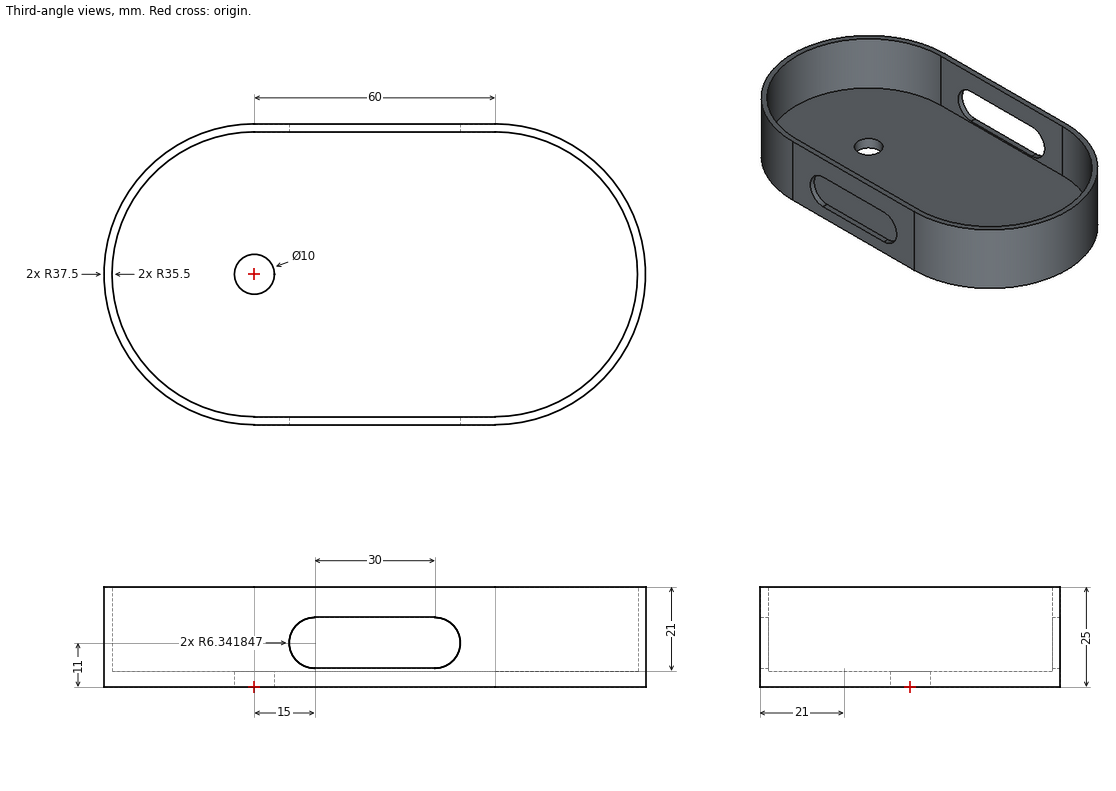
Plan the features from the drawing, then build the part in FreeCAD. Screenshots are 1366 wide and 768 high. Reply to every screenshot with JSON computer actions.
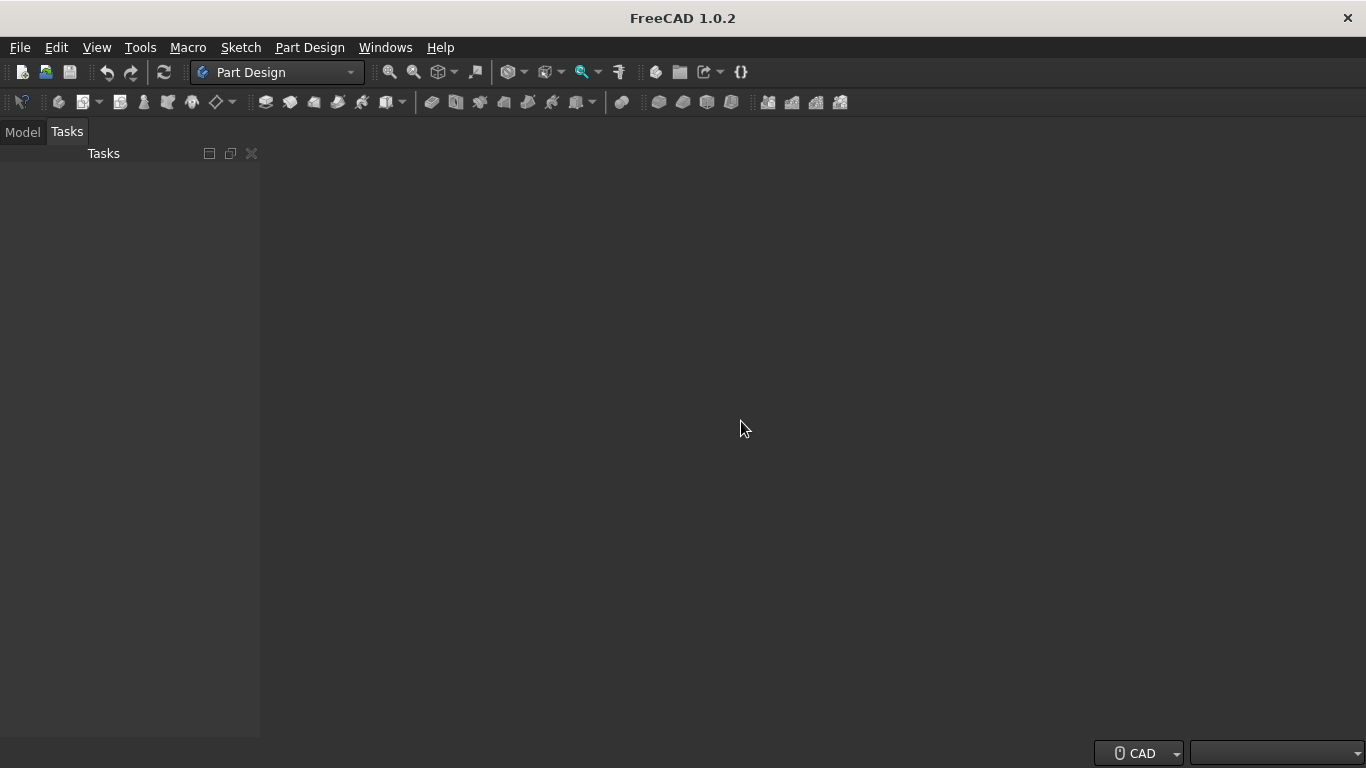
{"action": "left_click", "coordinate": [22, 72]}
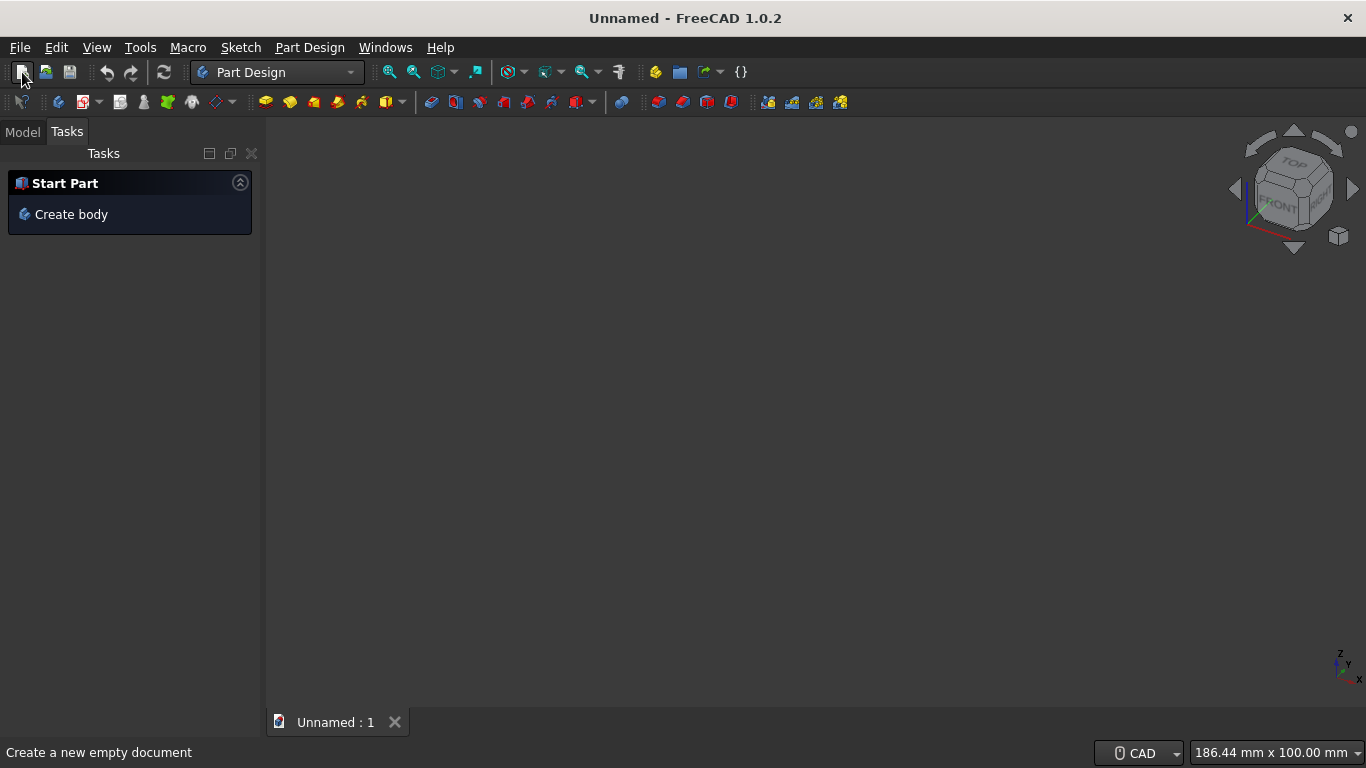
{"action": "left_click", "coordinate": [84, 102]}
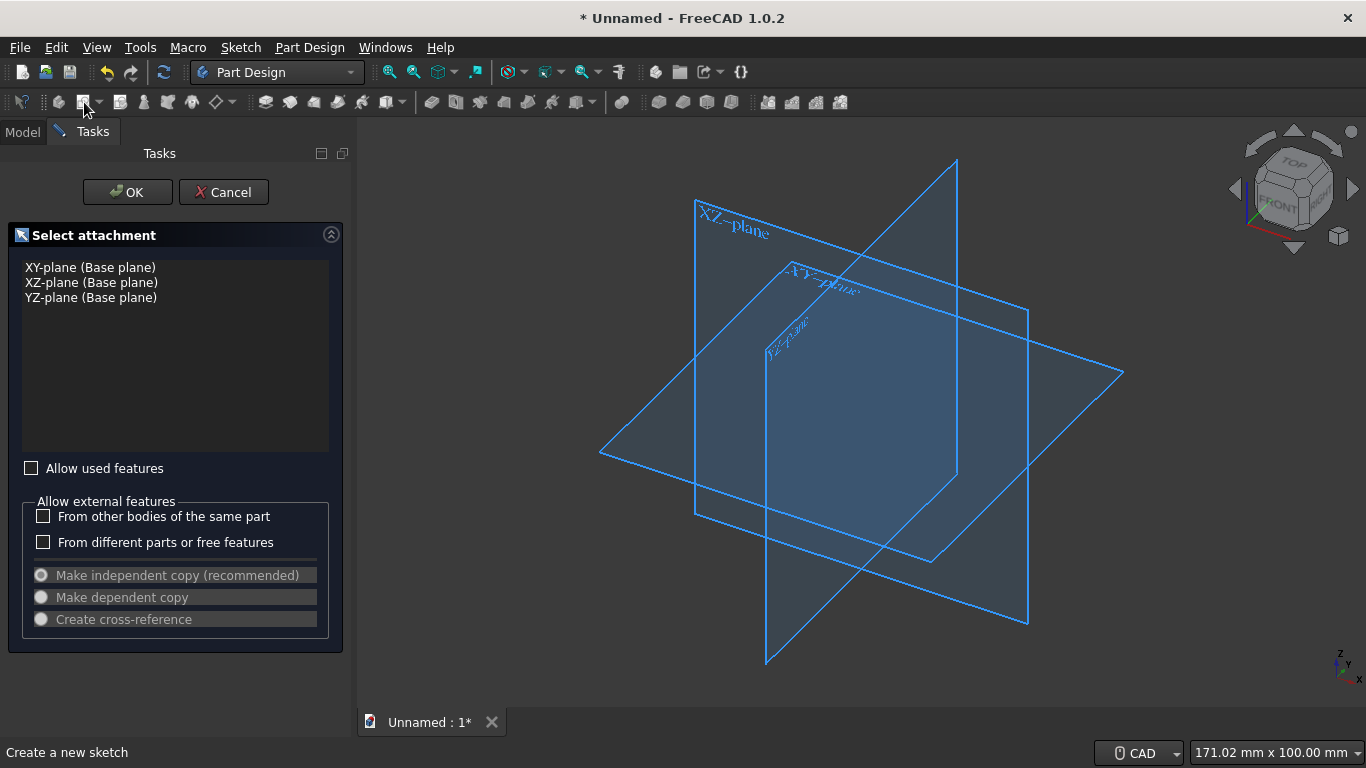
{"action": "left_click", "coordinate": [82, 268]}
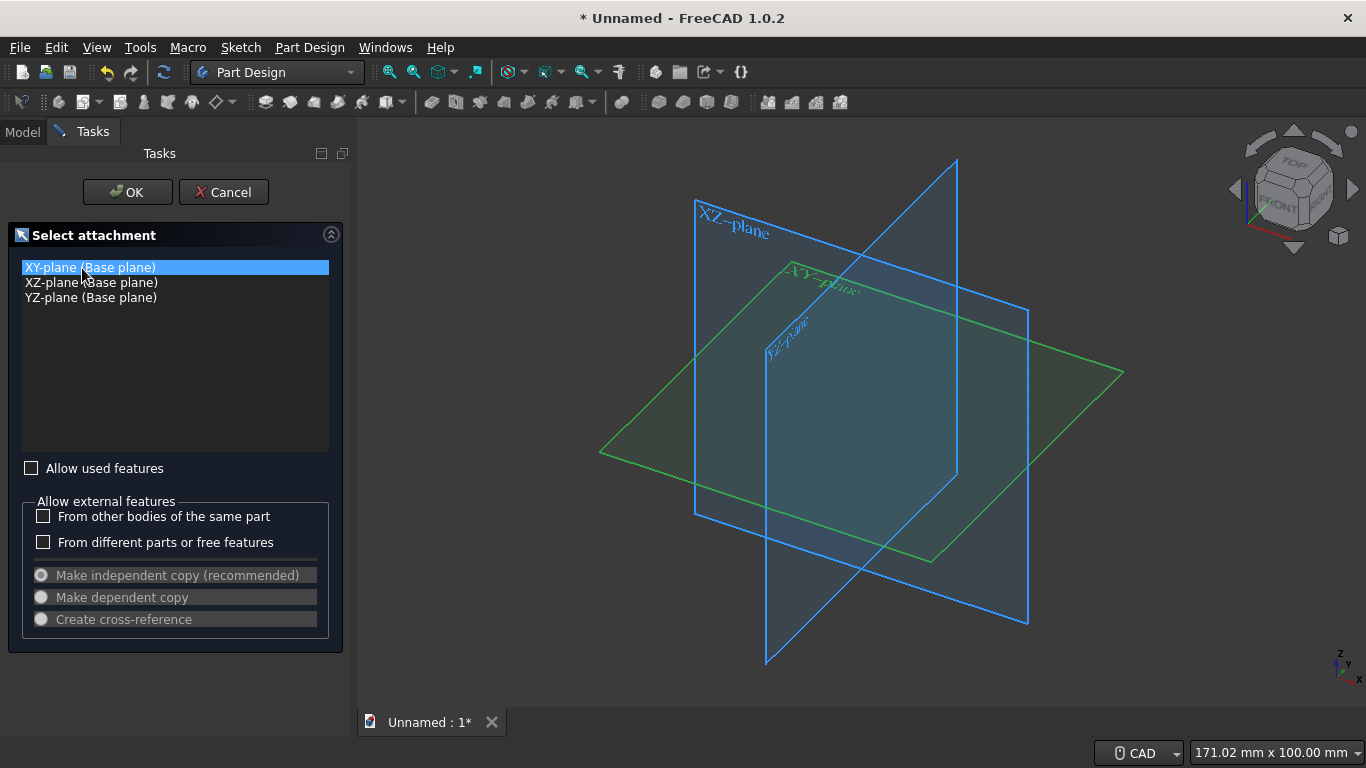
{"action": "left_click", "coordinate": [128, 192]}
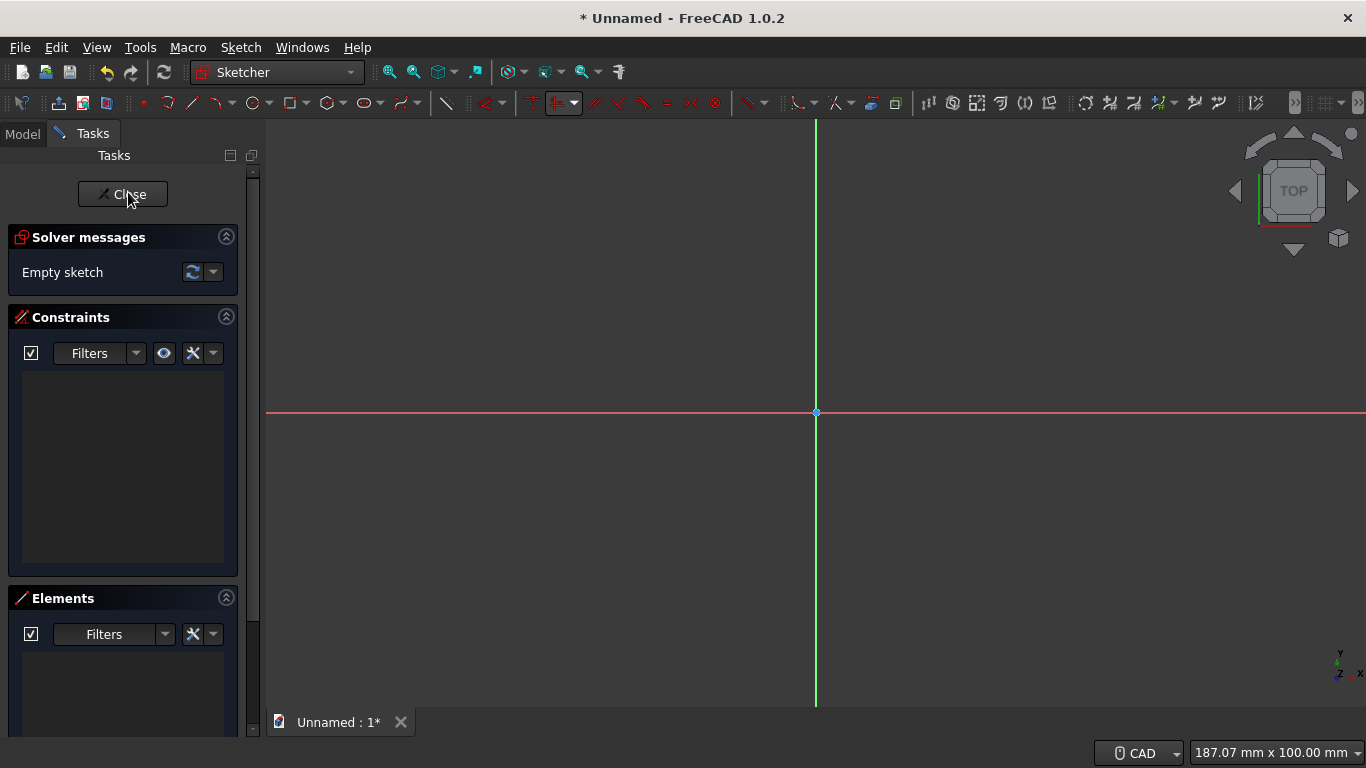
{"action": "scroll", "coordinate": [294, 413], "scroll_direction": "down", "scroll_amount": 2}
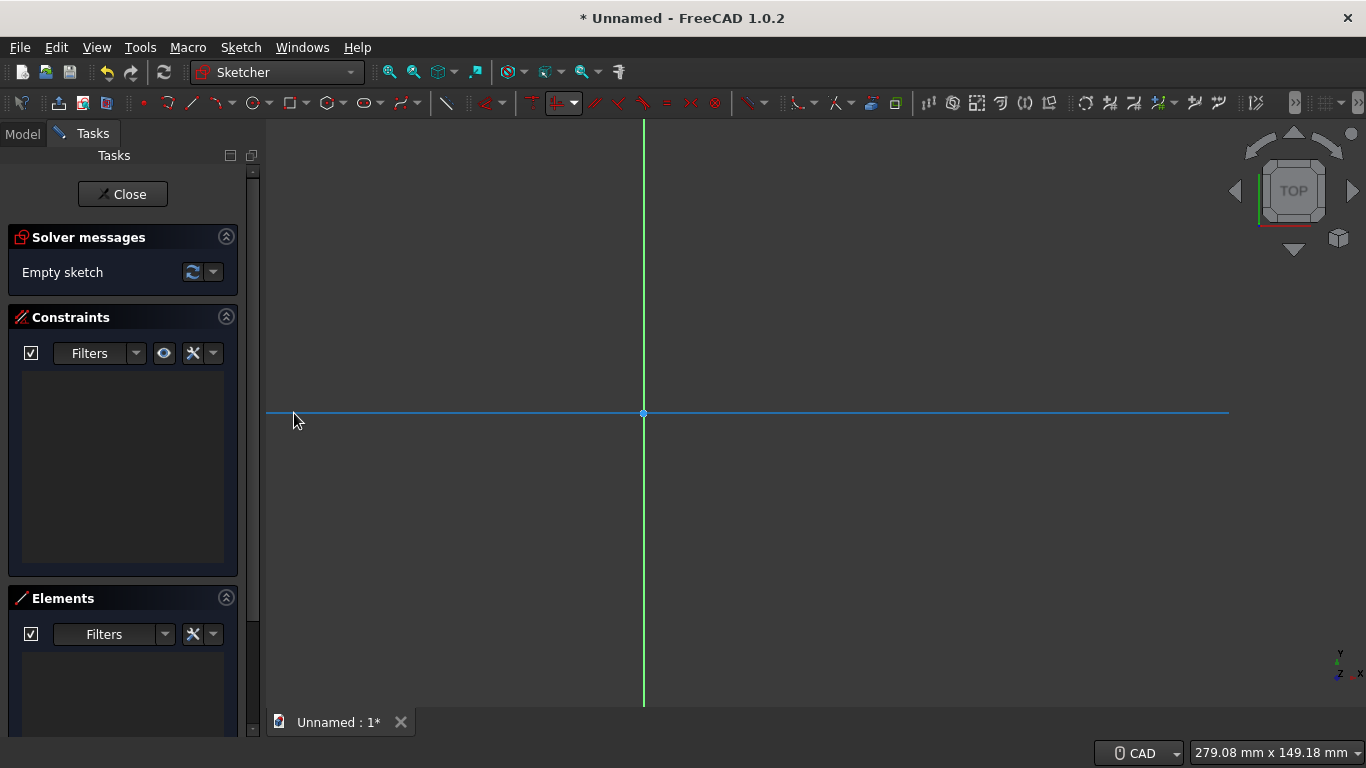
{"action": "left_click", "coordinate": [364, 104]}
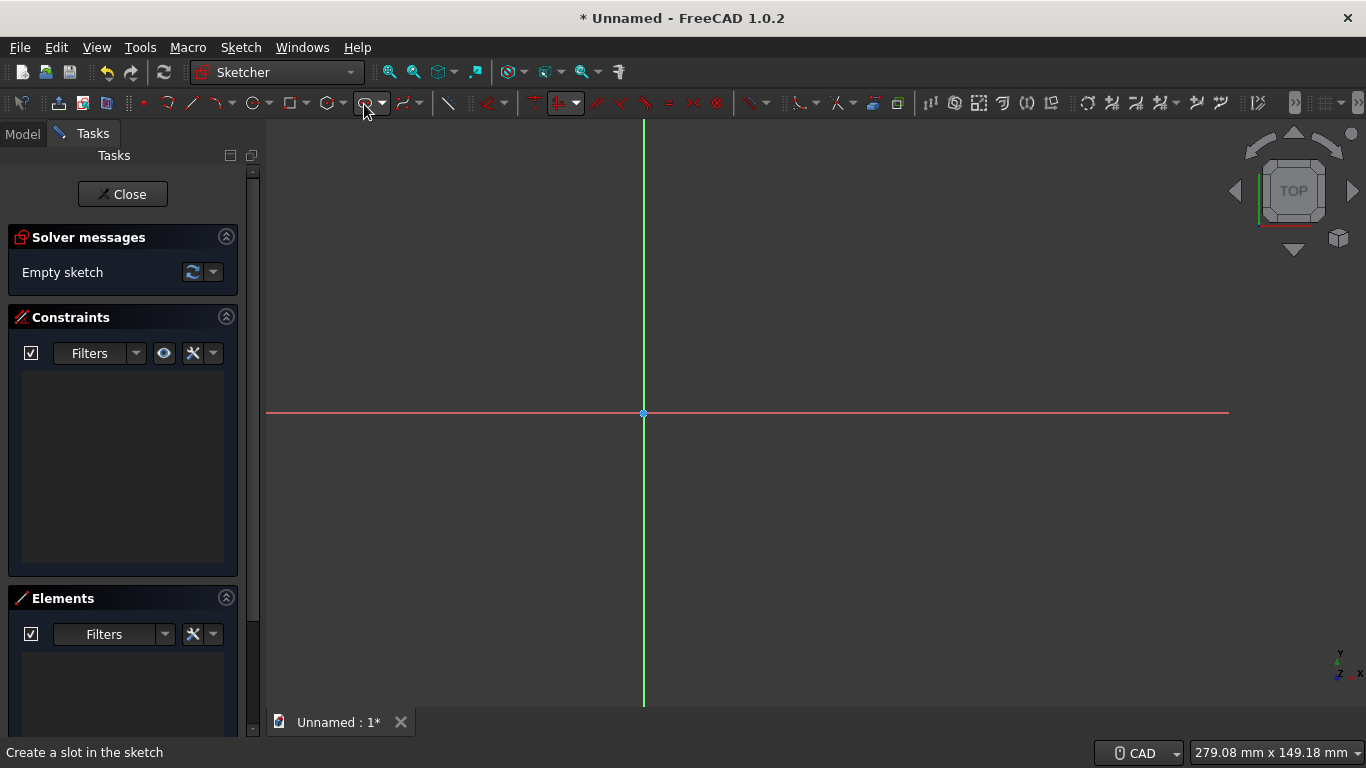
{"action": "left_click", "coordinate": [644, 413]}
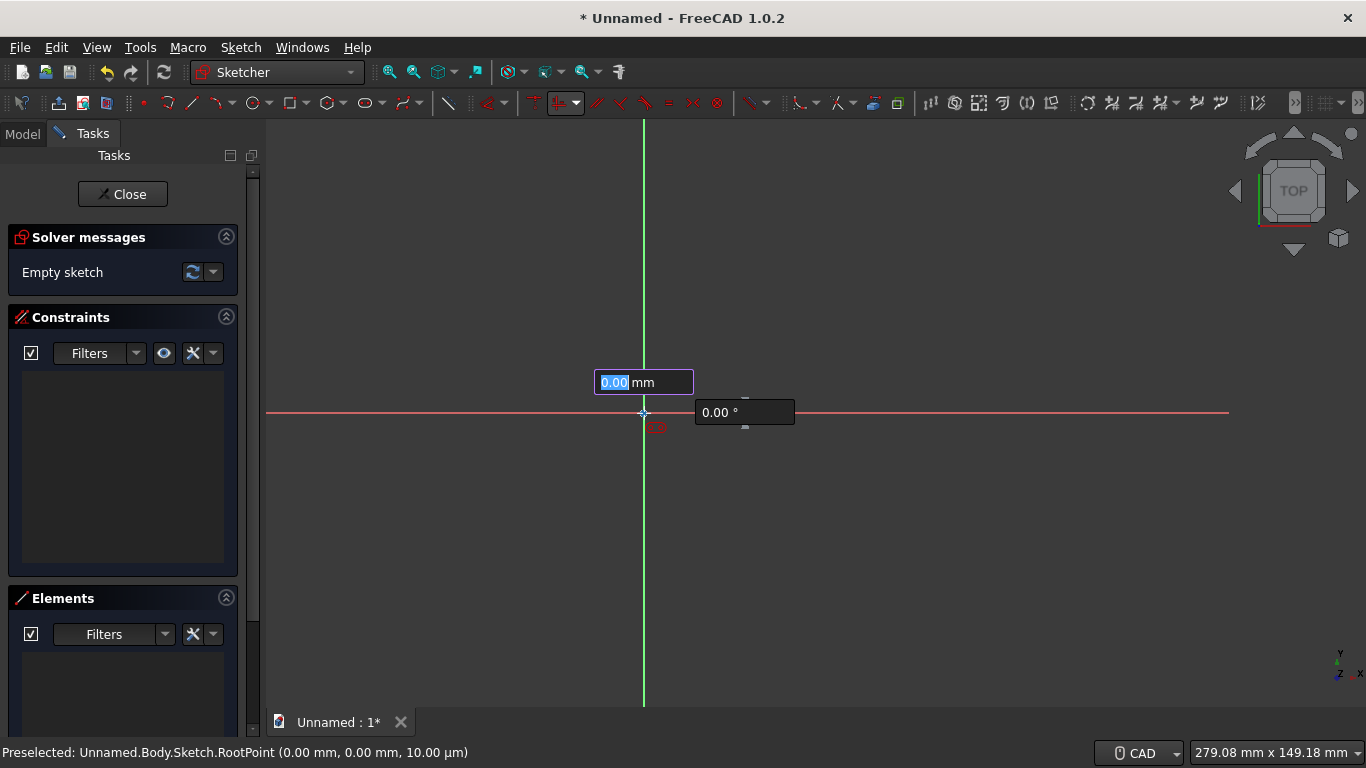
{"action": "left_click", "coordinate": [880, 404]}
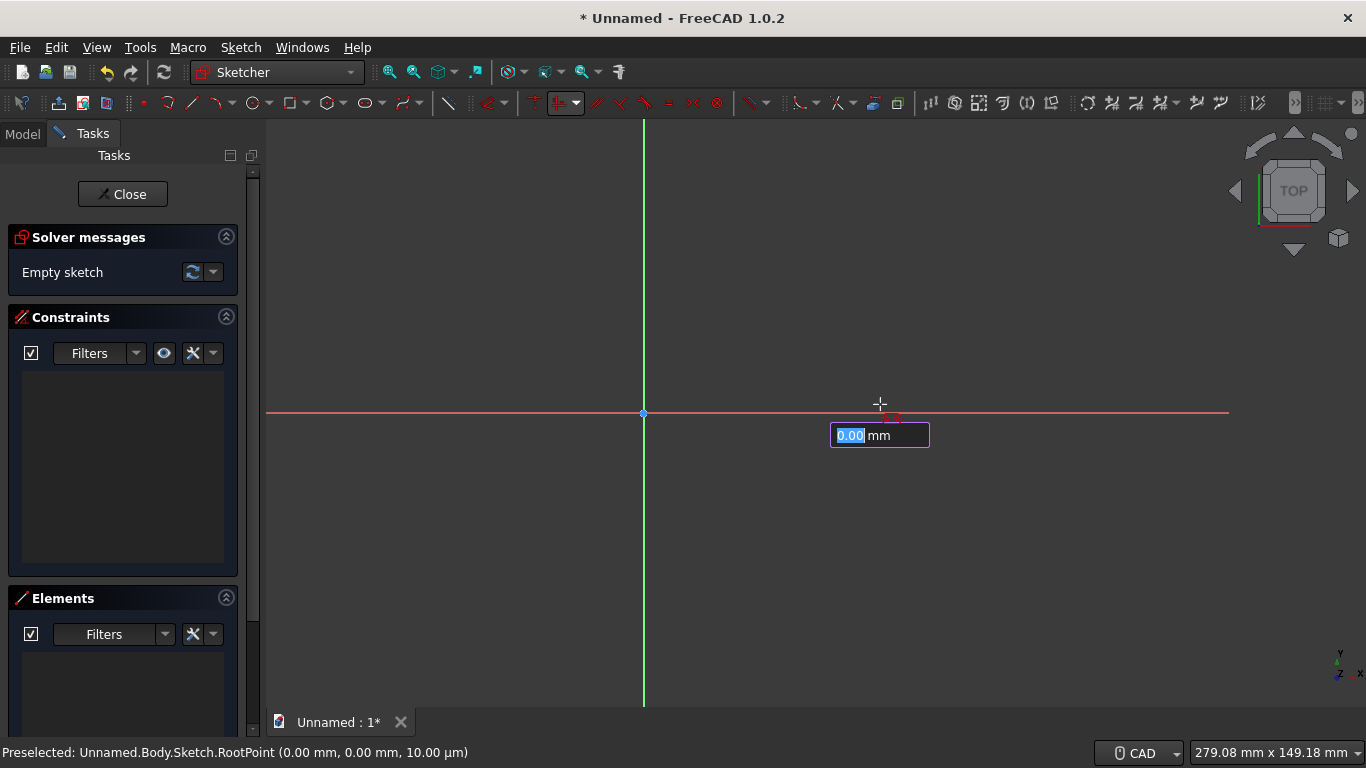
{"action": "left_click", "coordinate": [762, 265]}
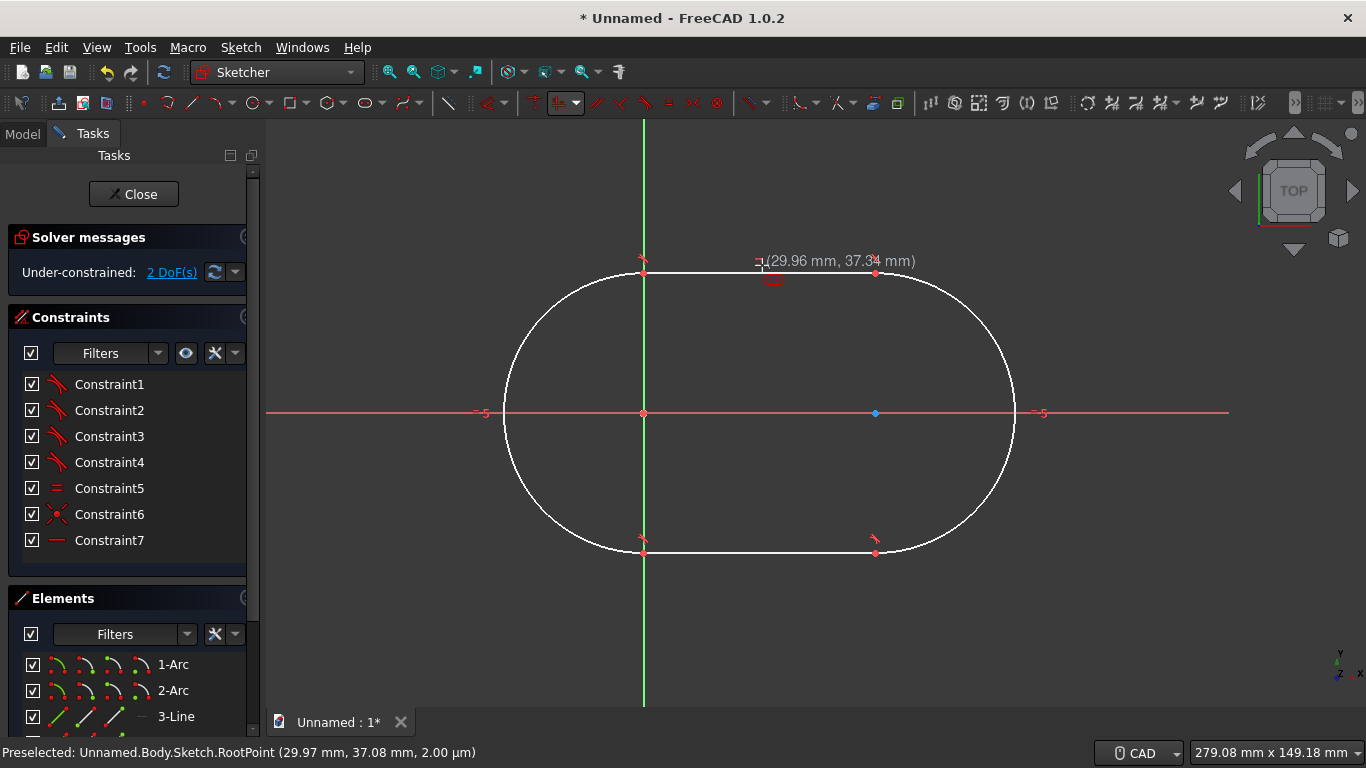
{"action": "left_click", "coordinate": [254, 104]}